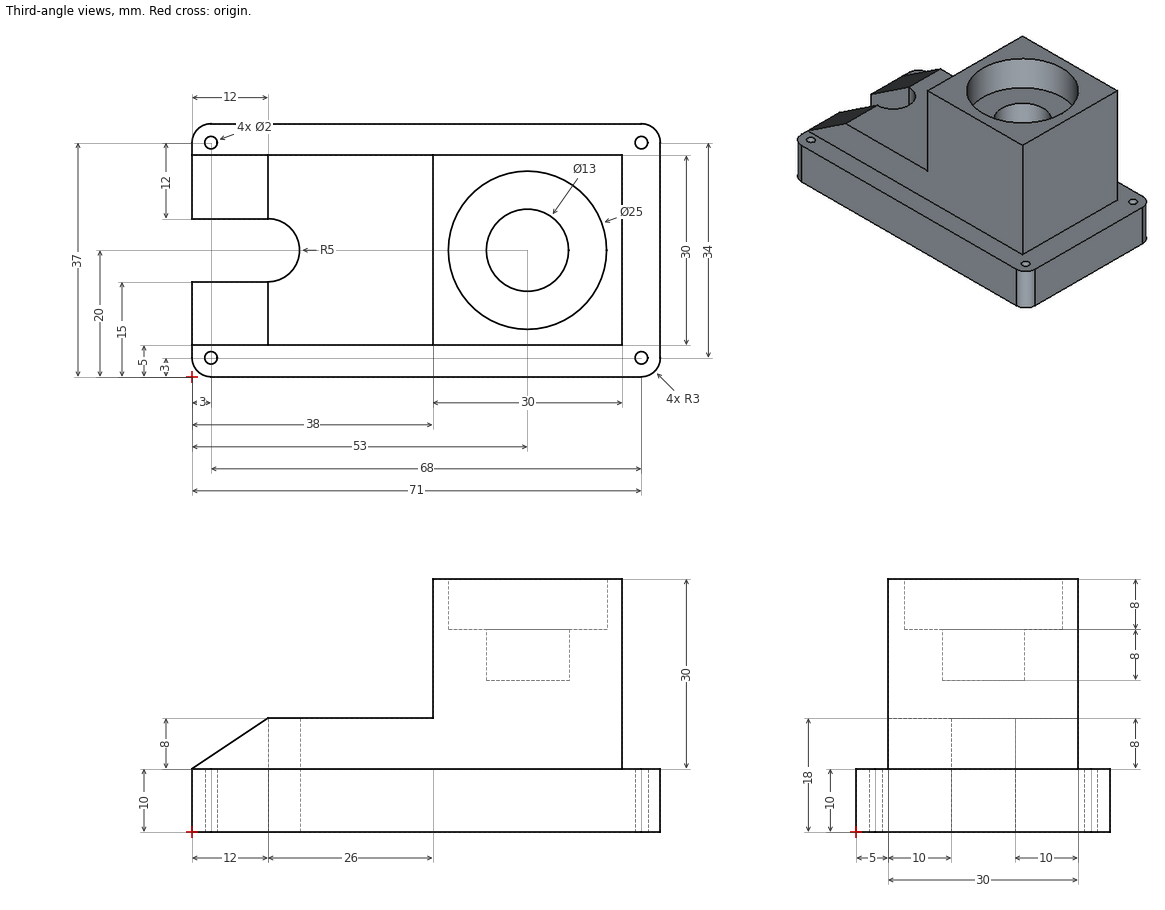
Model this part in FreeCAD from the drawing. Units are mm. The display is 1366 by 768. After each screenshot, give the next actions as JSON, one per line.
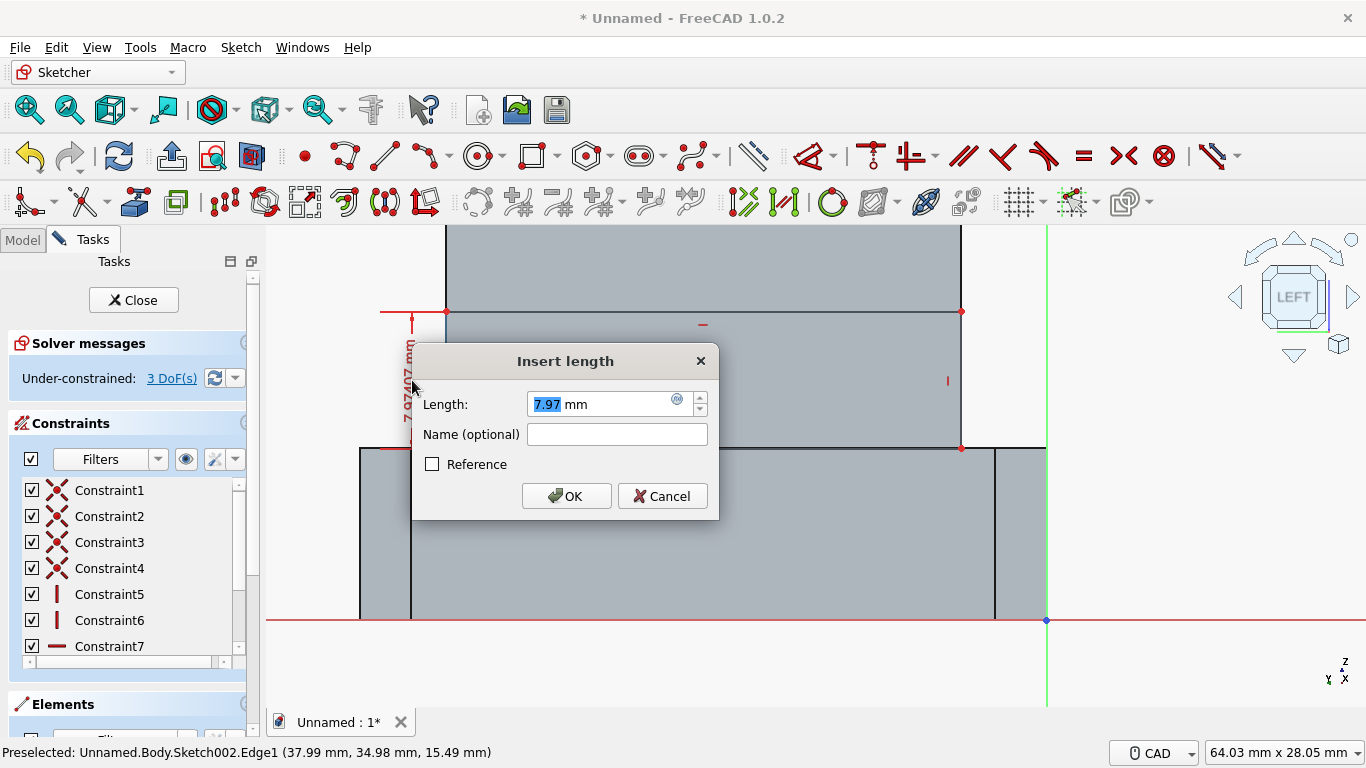
{"action": "type", "text": "8"}
{"action": "key", "text": "Return"}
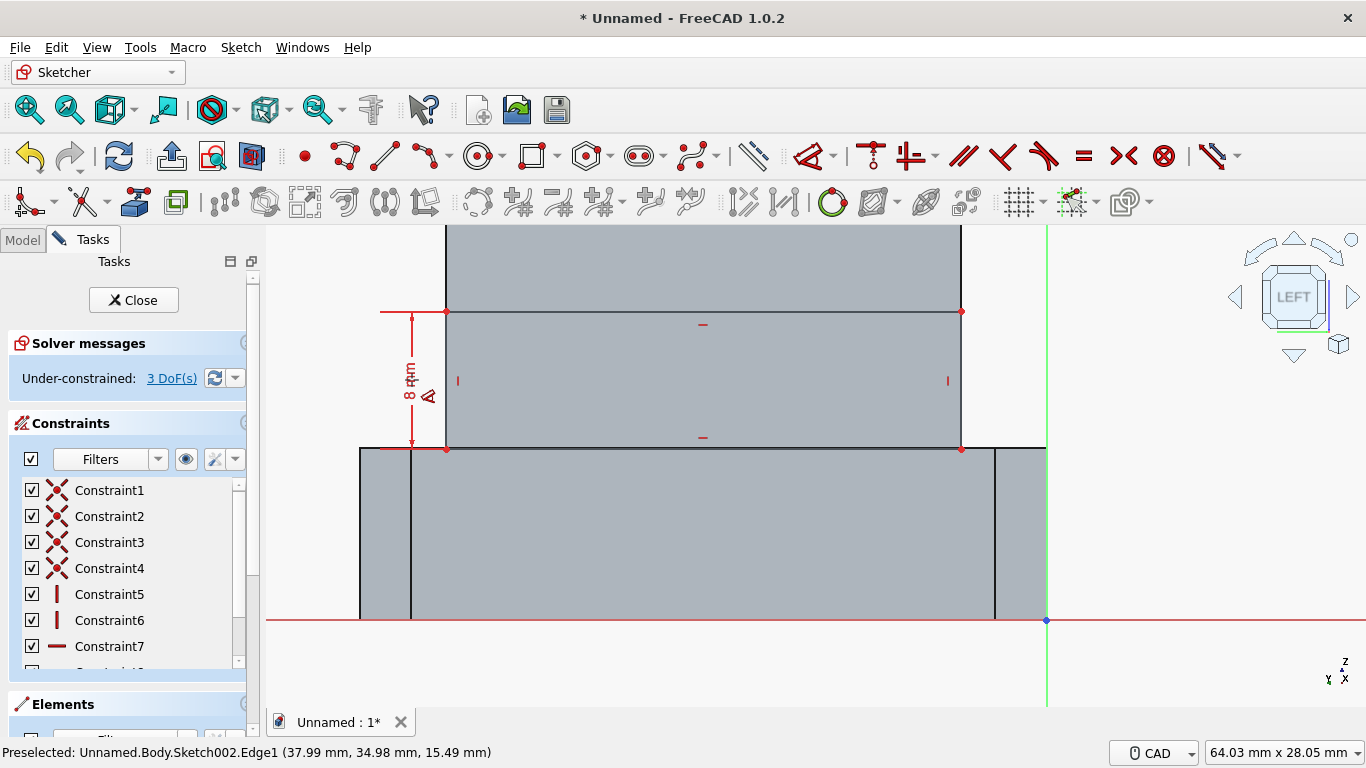
{"action": "left_click", "coordinate": [601, 449]}
{"action": "left_click", "coordinate": [704, 415]}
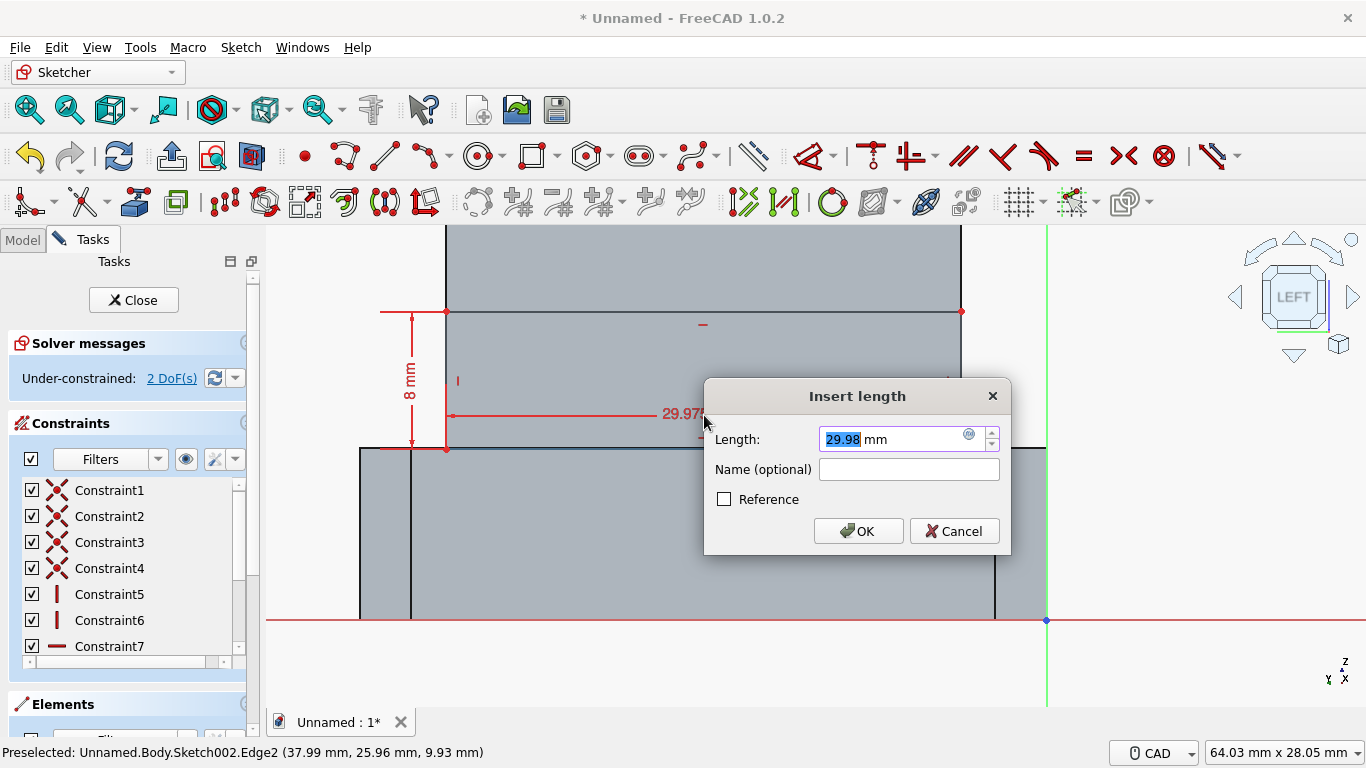
{"action": "type", "text": "30"}
{"action": "key", "text": "Return"}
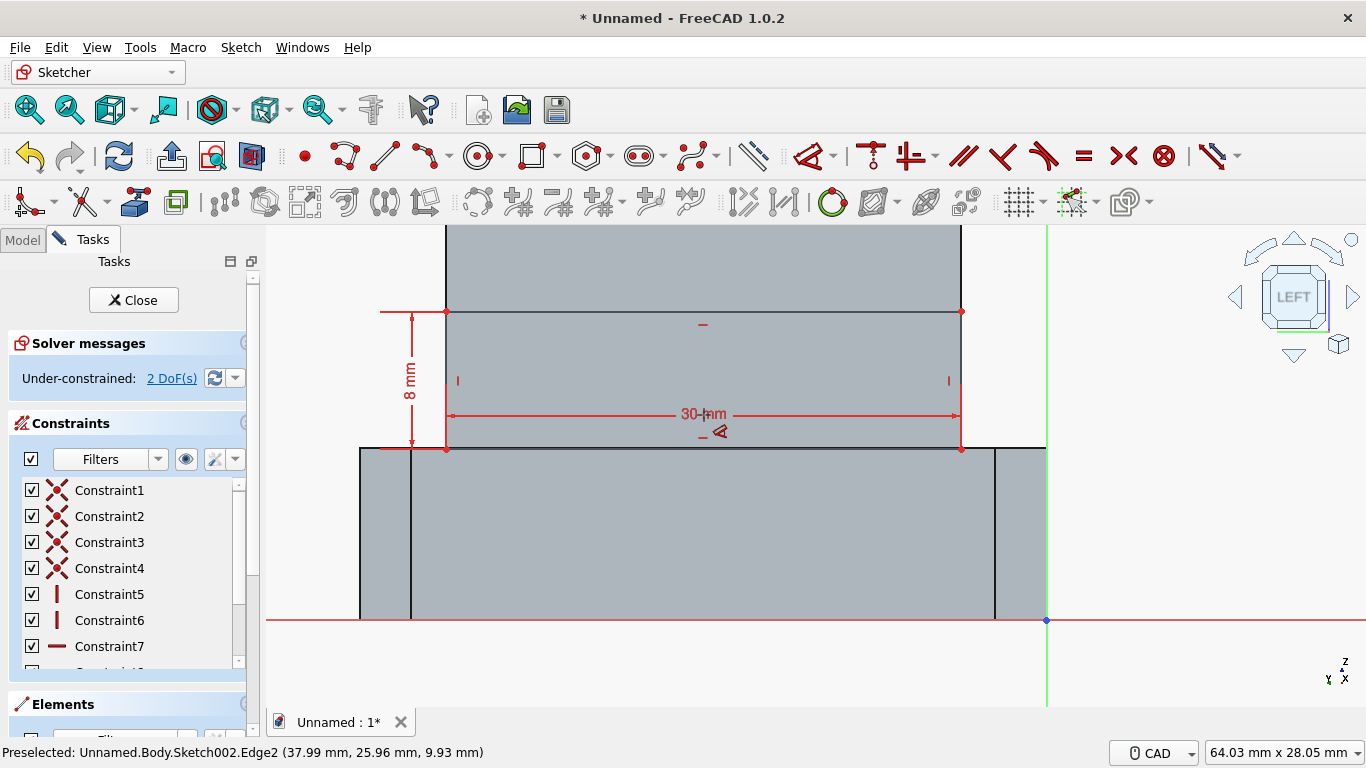
{"action": "left_click", "coordinate": [961, 449]}
{"action": "left_click", "coordinate": [1004, 654]}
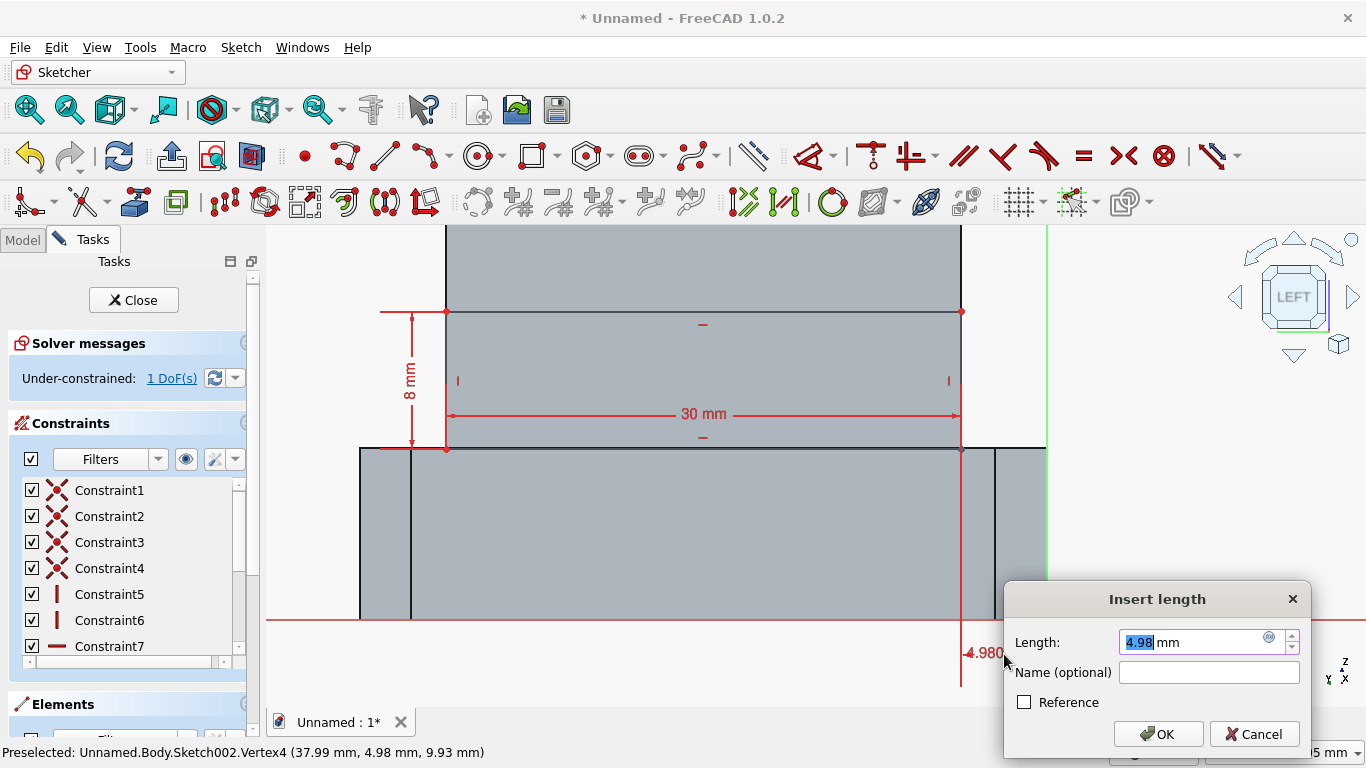
{"action": "type", "text": "5"}
{"action": "key", "text": "Return"}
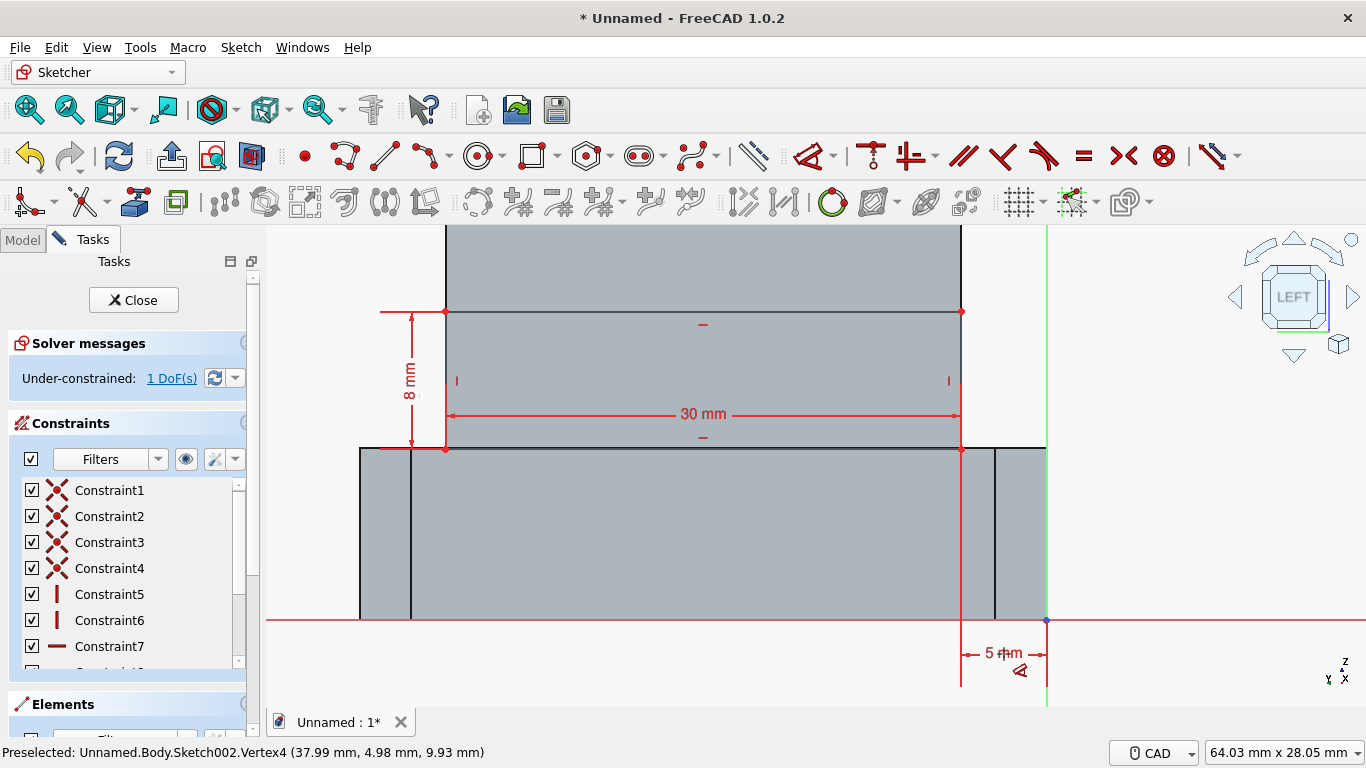
{"action": "left_click", "coordinate": [446, 312]}
{"action": "left_click", "coordinate": [1081, 466]}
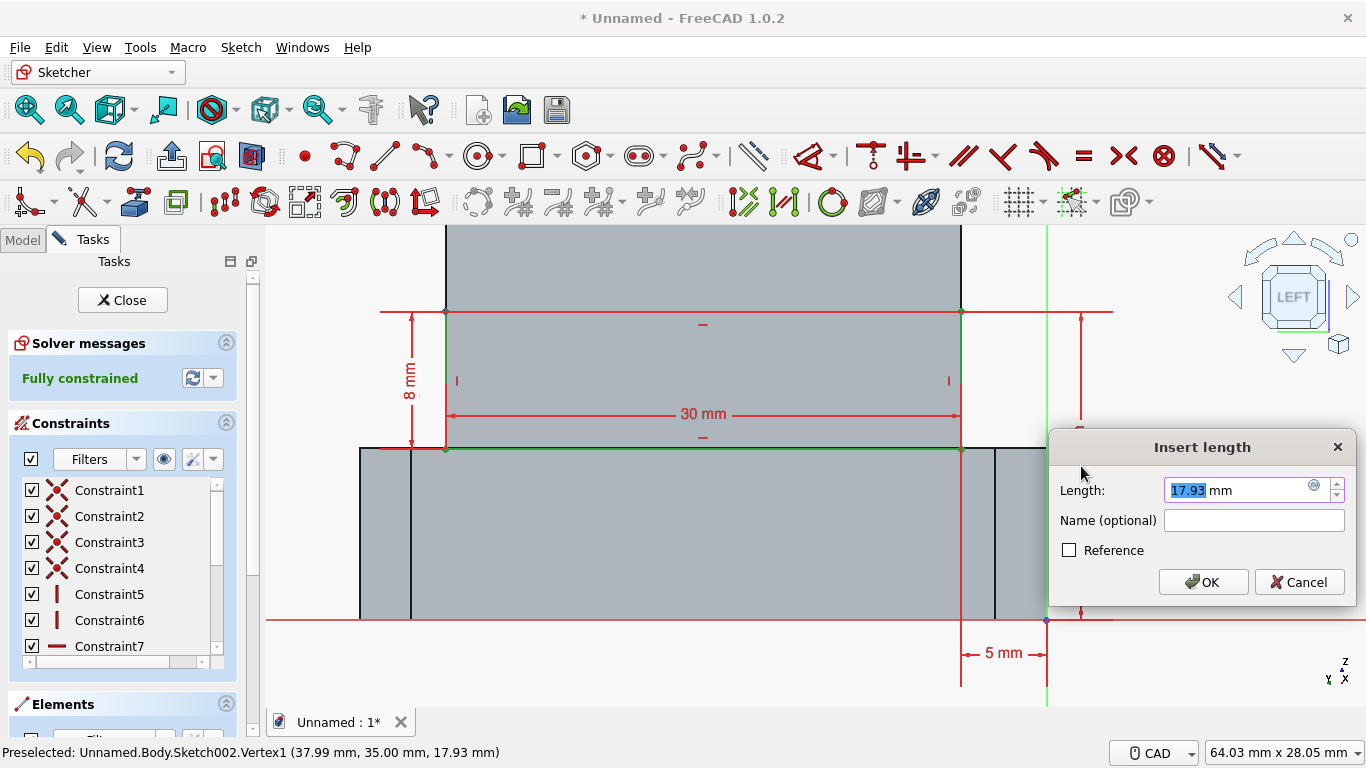
{"action": "type", "text": "18"}
{"action": "key", "text": "Return"}
{"action": "key", "text": "Escape"}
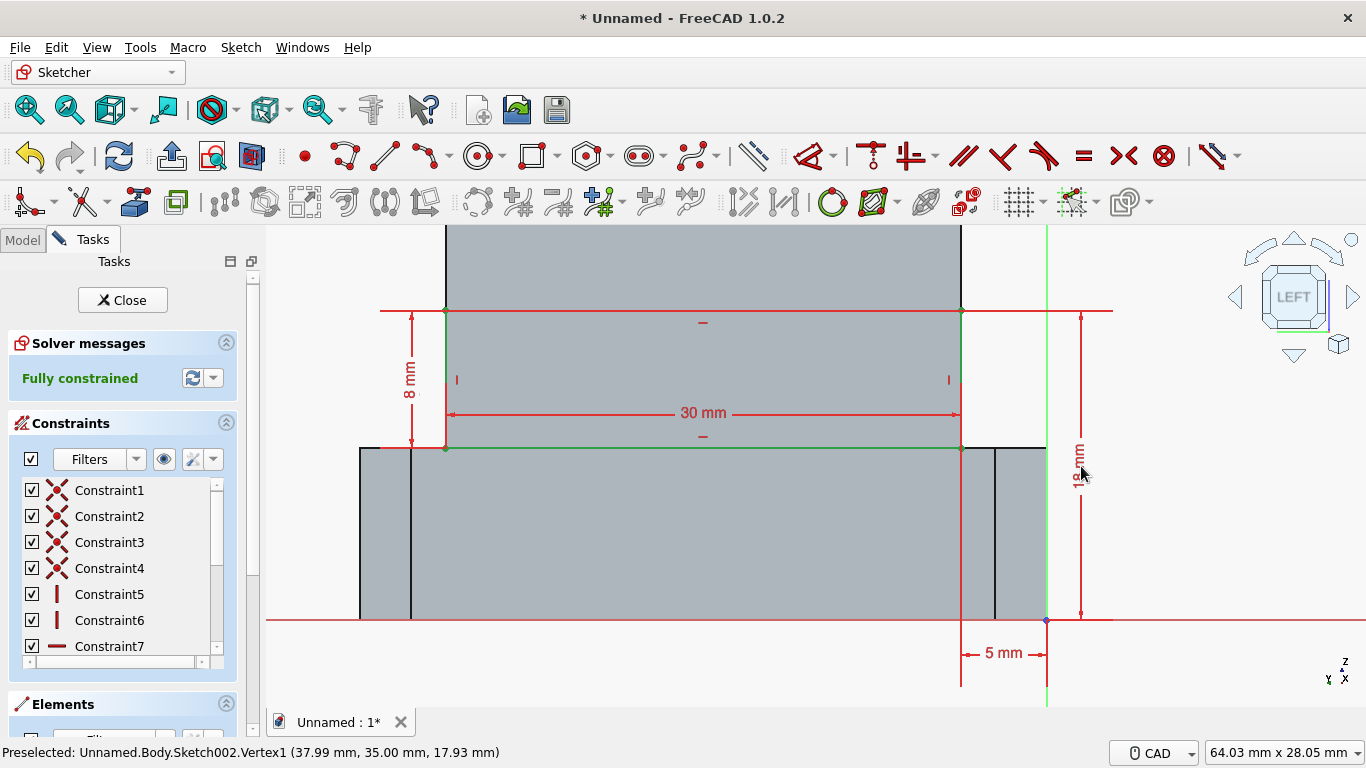
{"action": "left_click", "coordinate": [123, 300]}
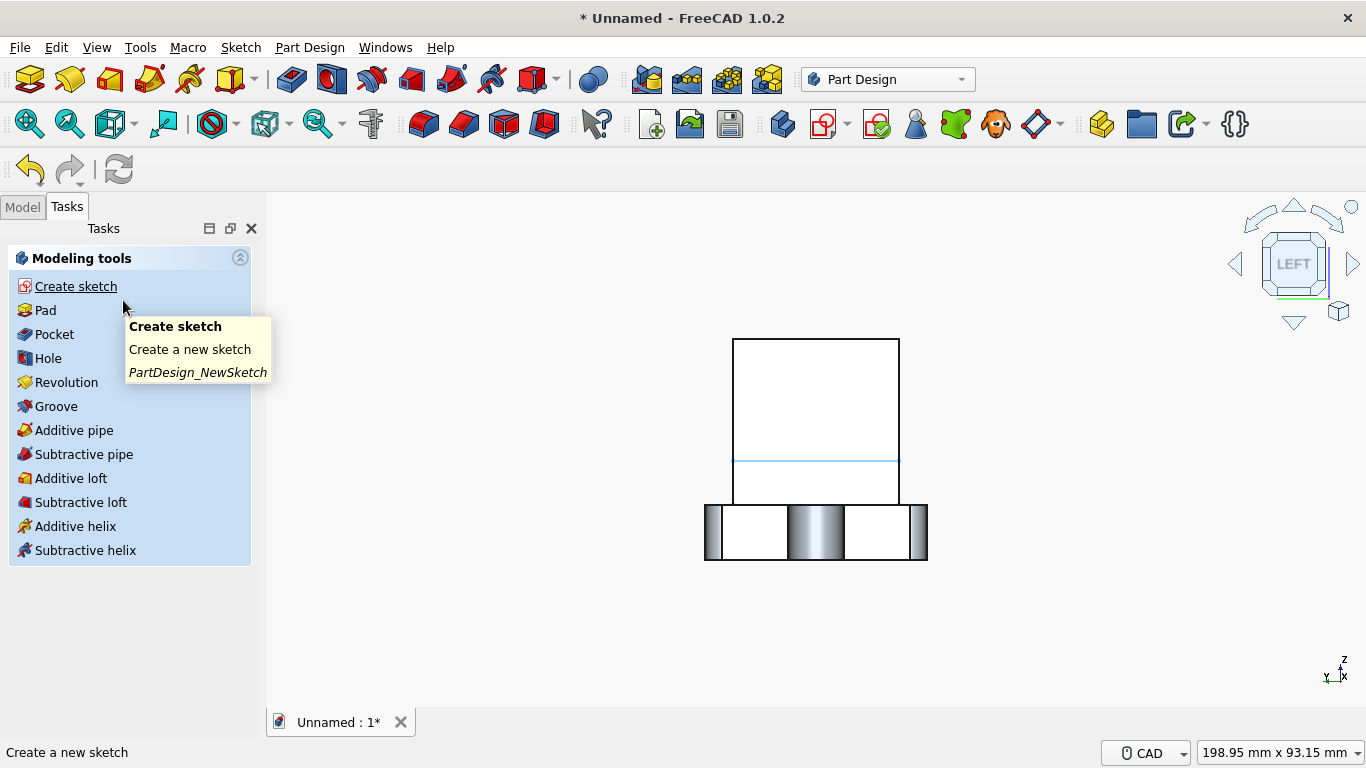
{"action": "left_click", "coordinate": [30, 80]}